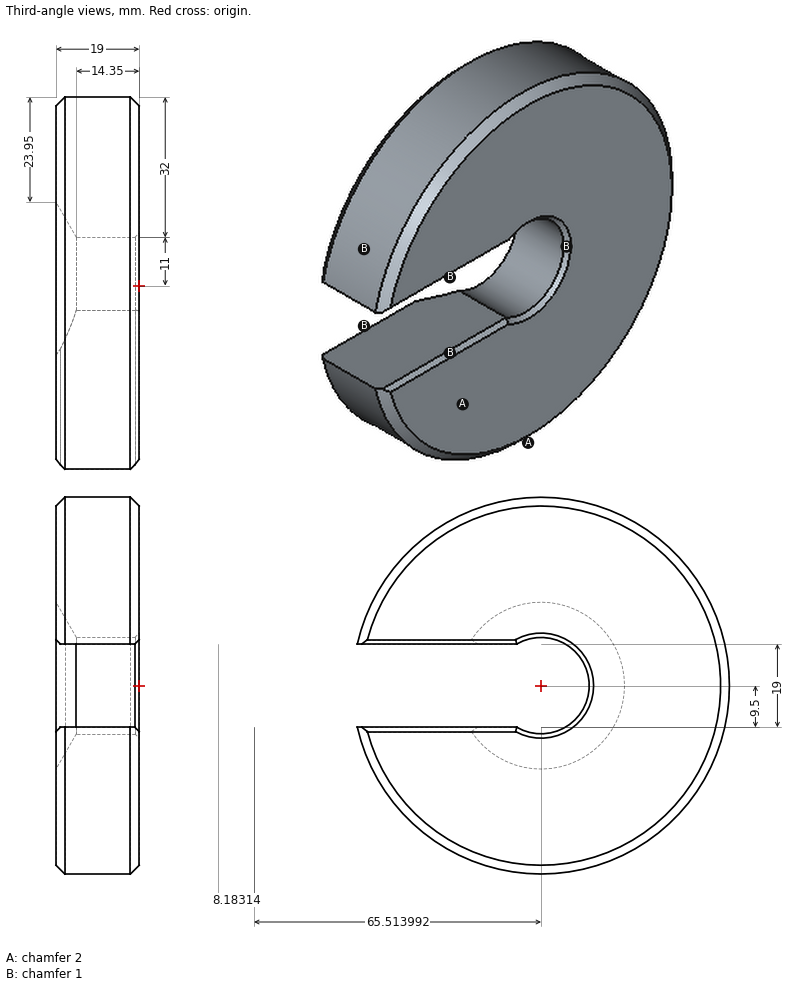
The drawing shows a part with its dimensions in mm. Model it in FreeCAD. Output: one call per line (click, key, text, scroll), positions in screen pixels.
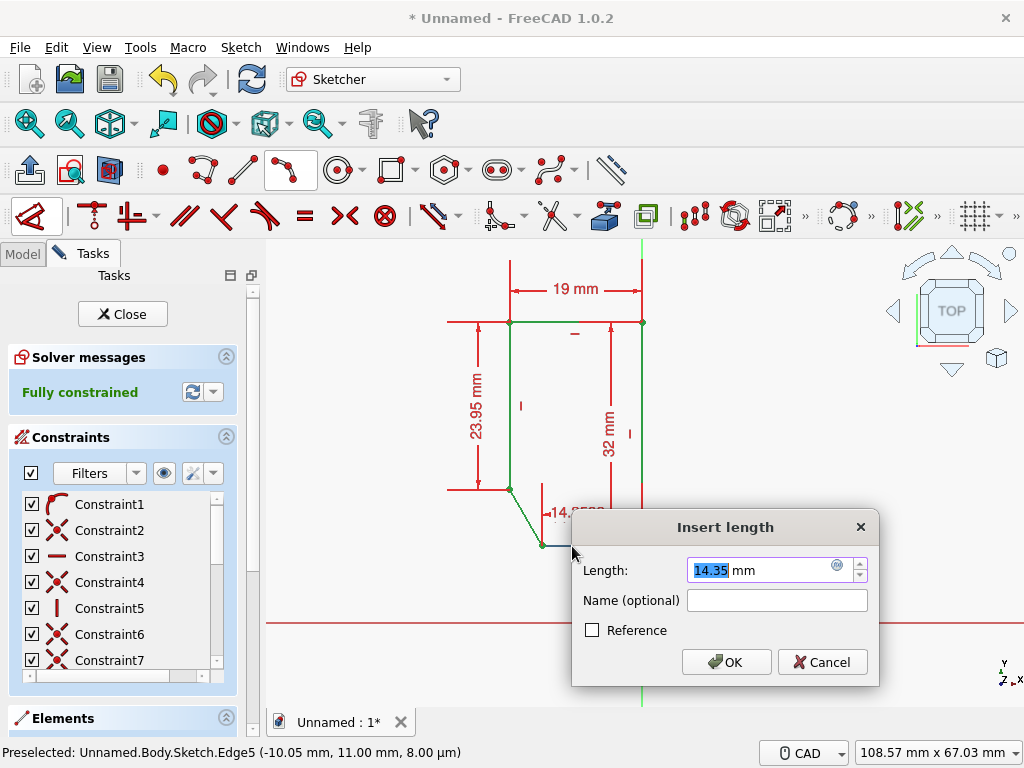
text(14.35)
key(Return)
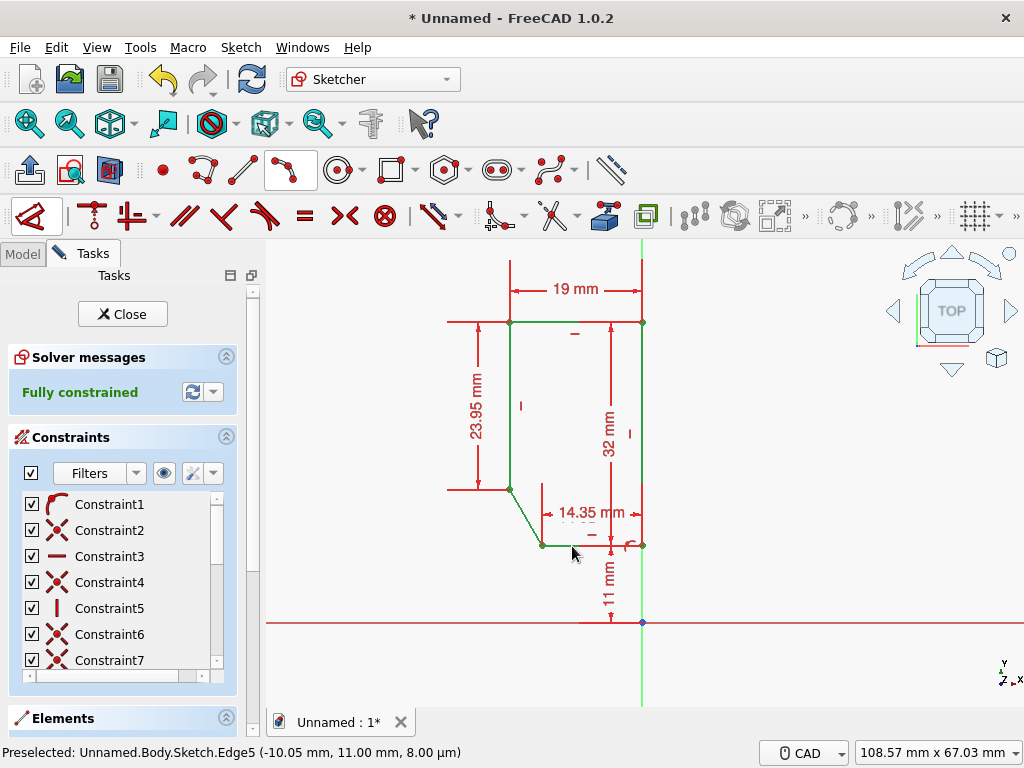
click(123, 314)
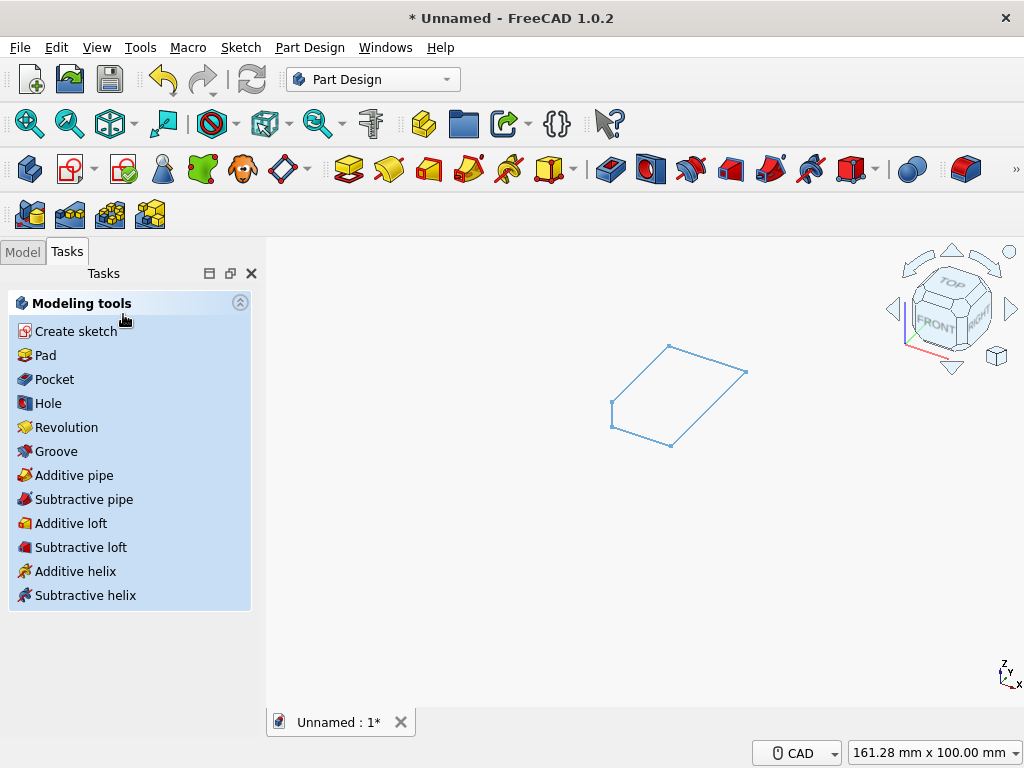
click(390, 170)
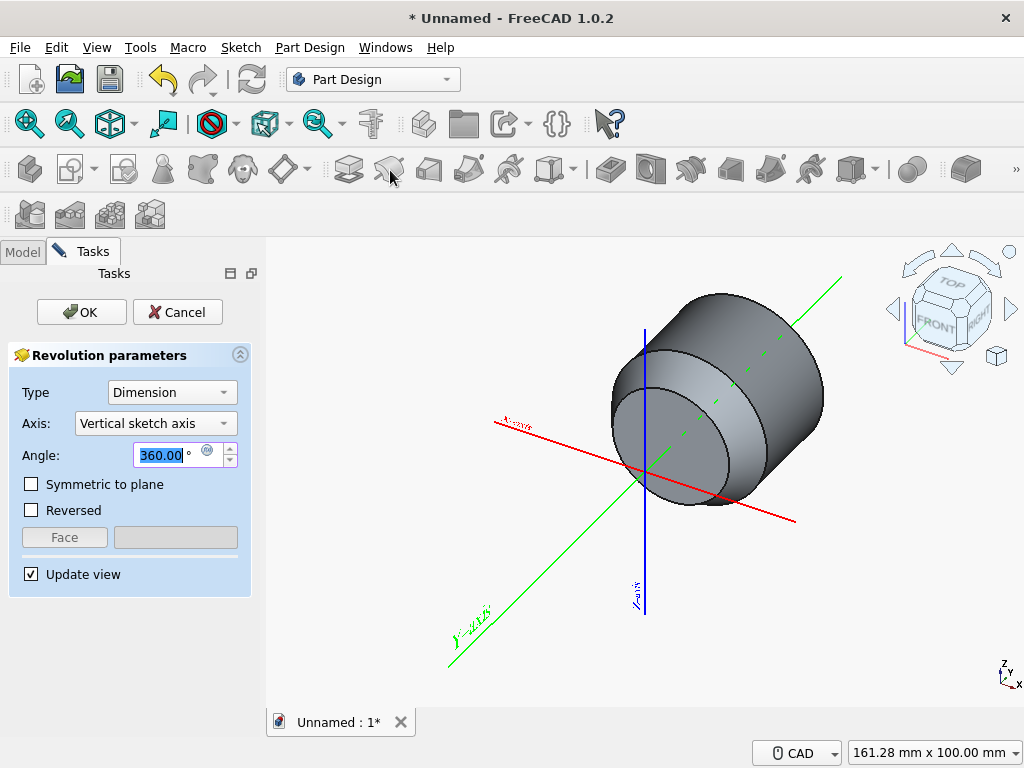
click(156, 424)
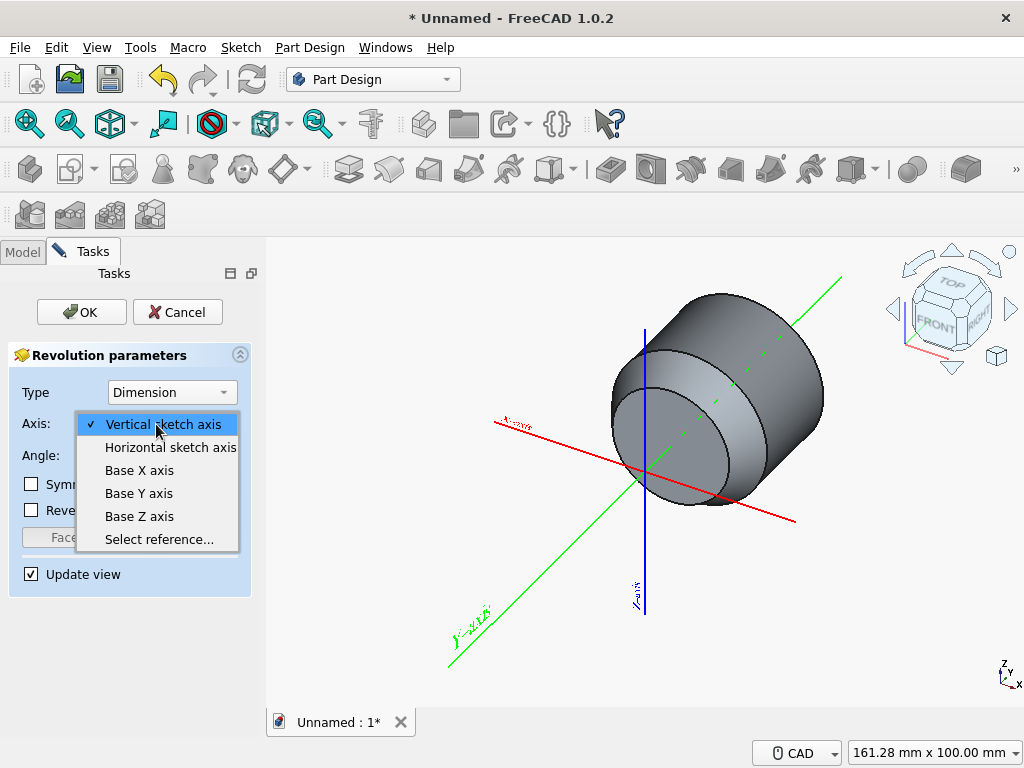
click(156, 448)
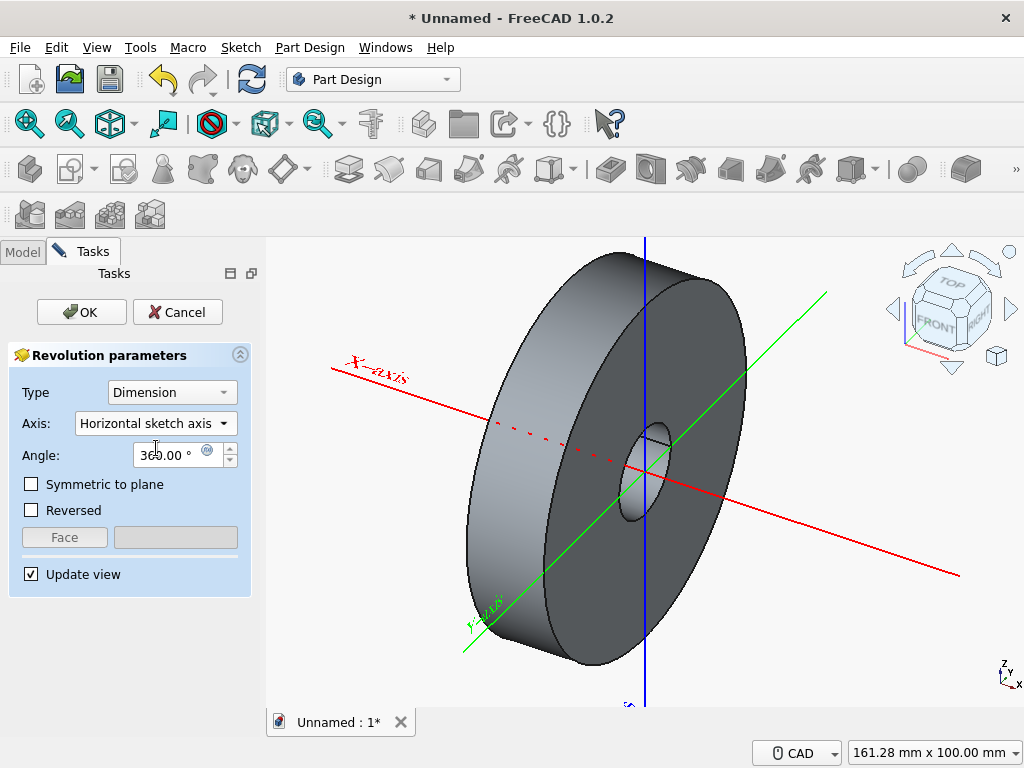
click(82, 312)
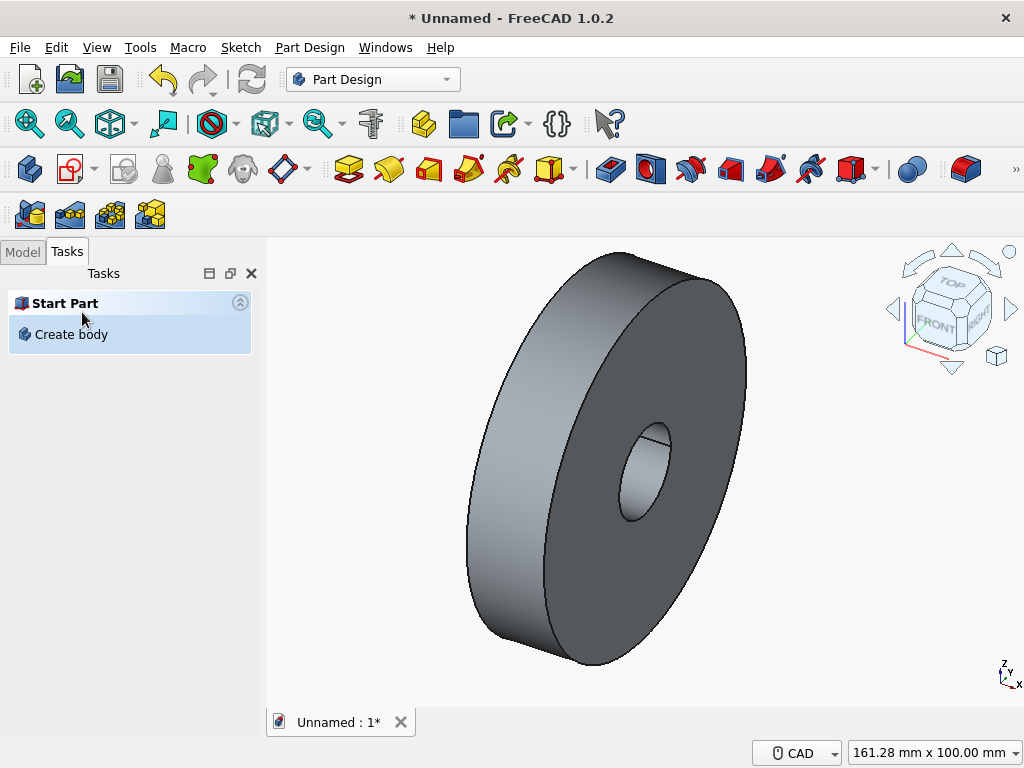
click(30, 124)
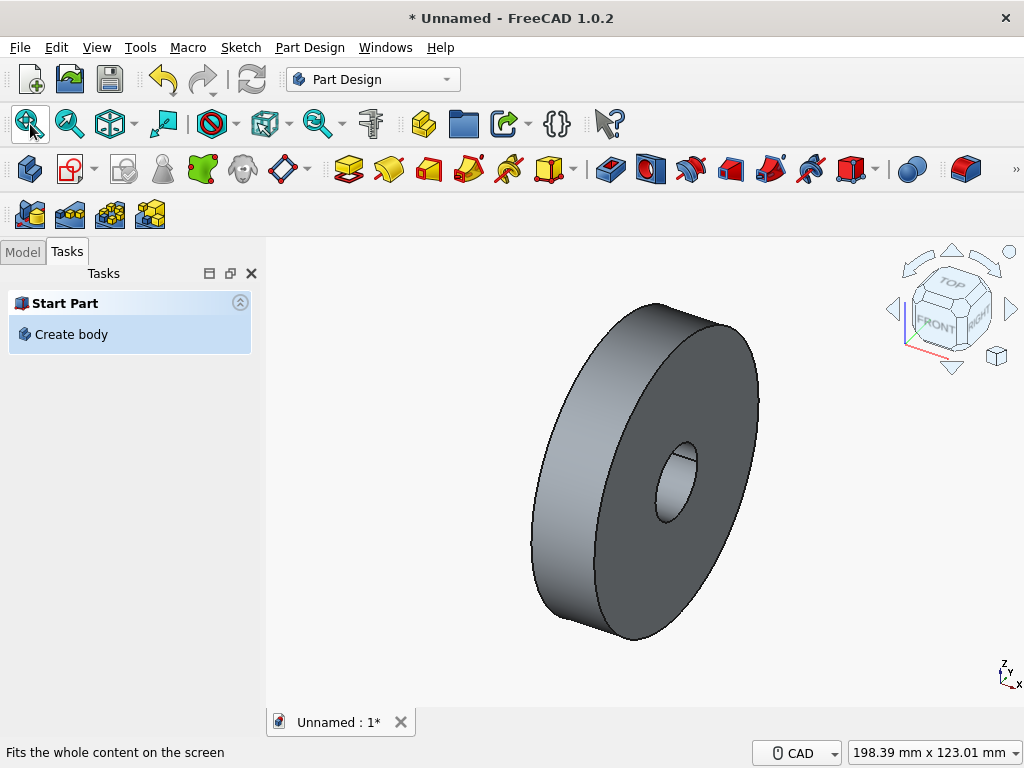
click(594, 563)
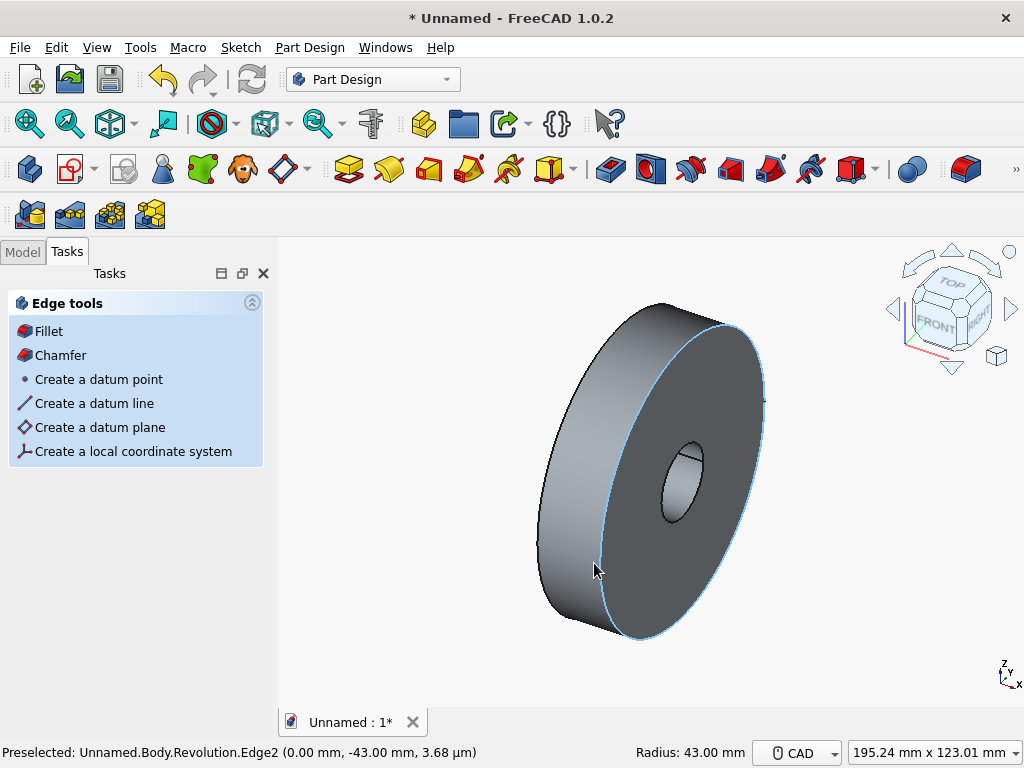
key(0)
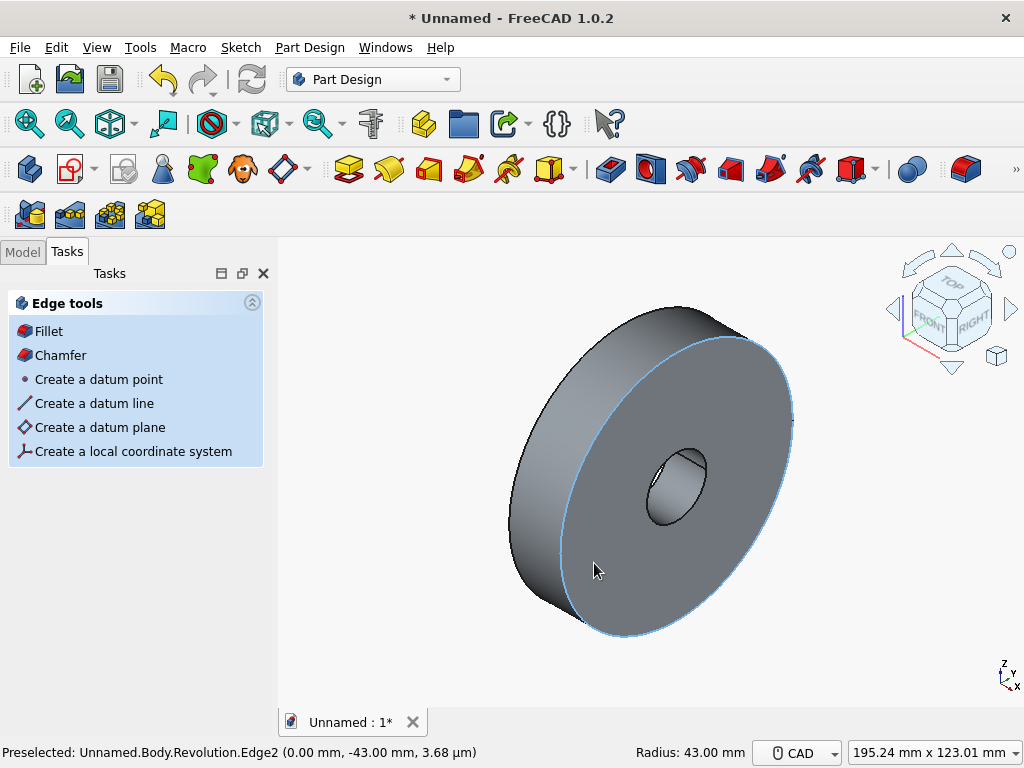
key(2)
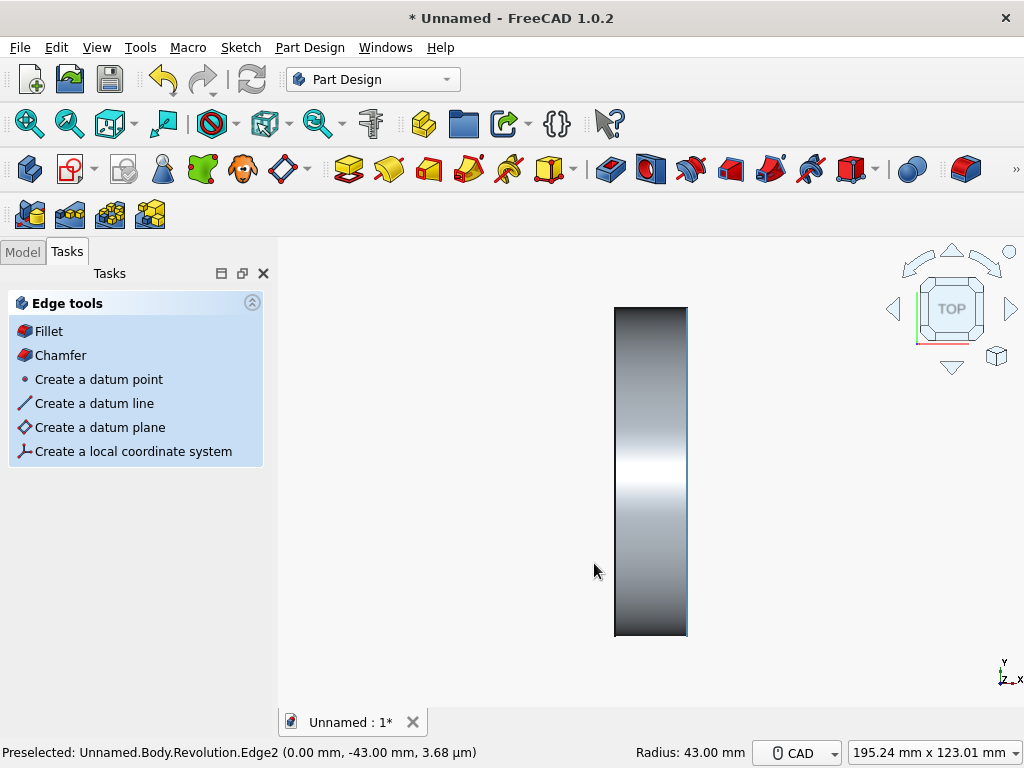
click(615, 604, ctrl)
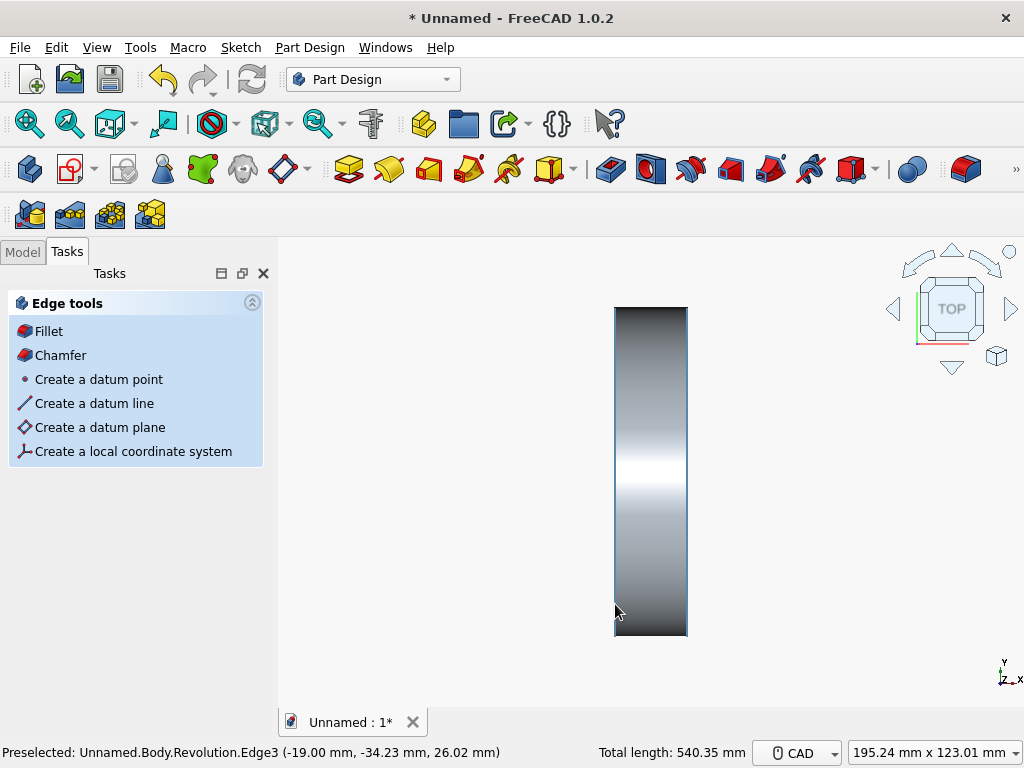
click(136, 355)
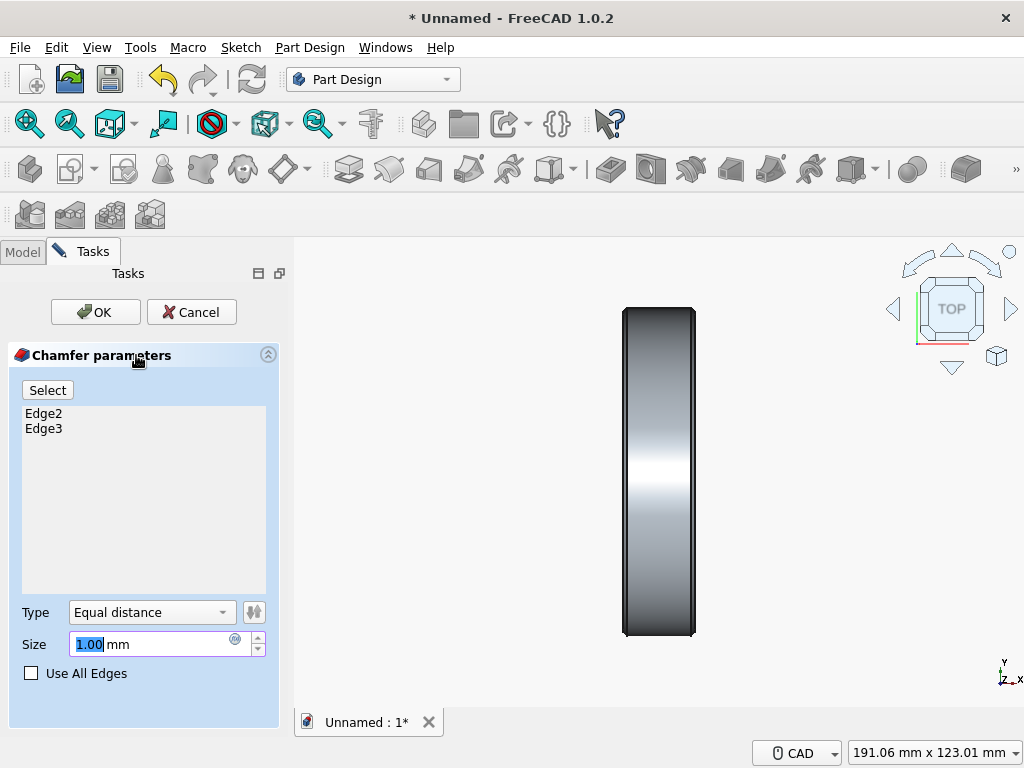
text(2)
key(Tab)